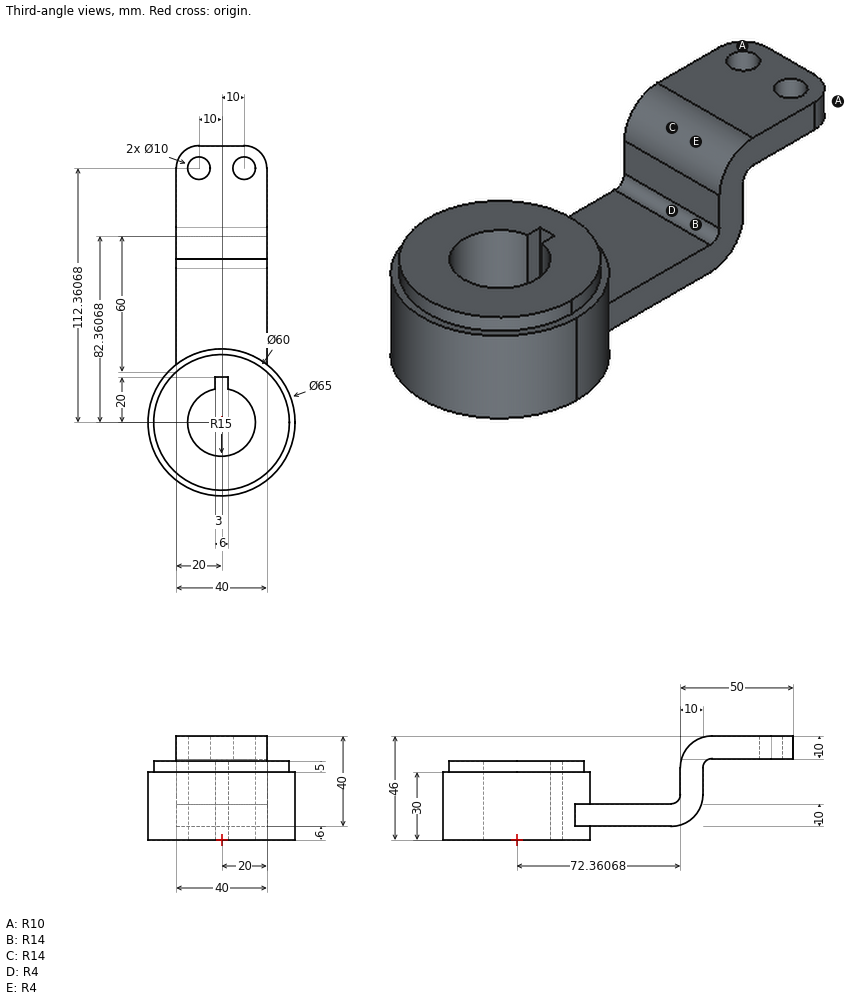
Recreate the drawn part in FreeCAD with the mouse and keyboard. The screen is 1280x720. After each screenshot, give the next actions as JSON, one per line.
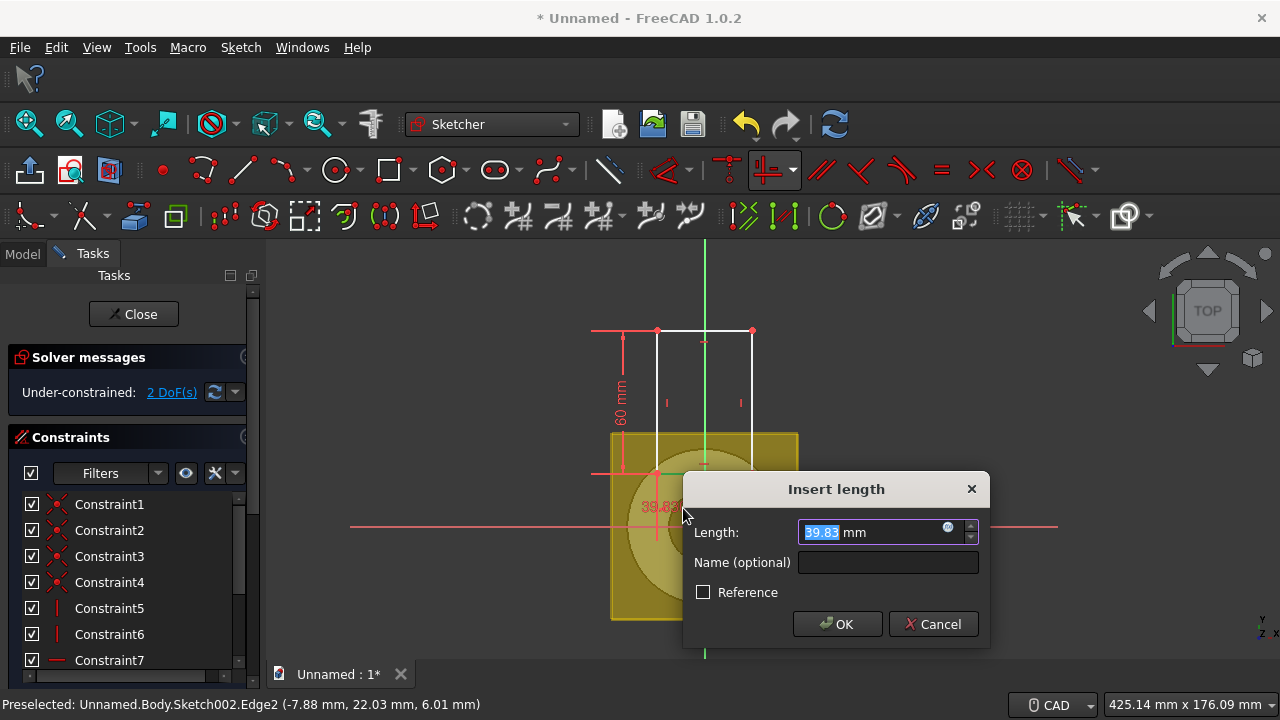
{"action": "type", "text": "40"}
{"action": "key", "text": "Return"}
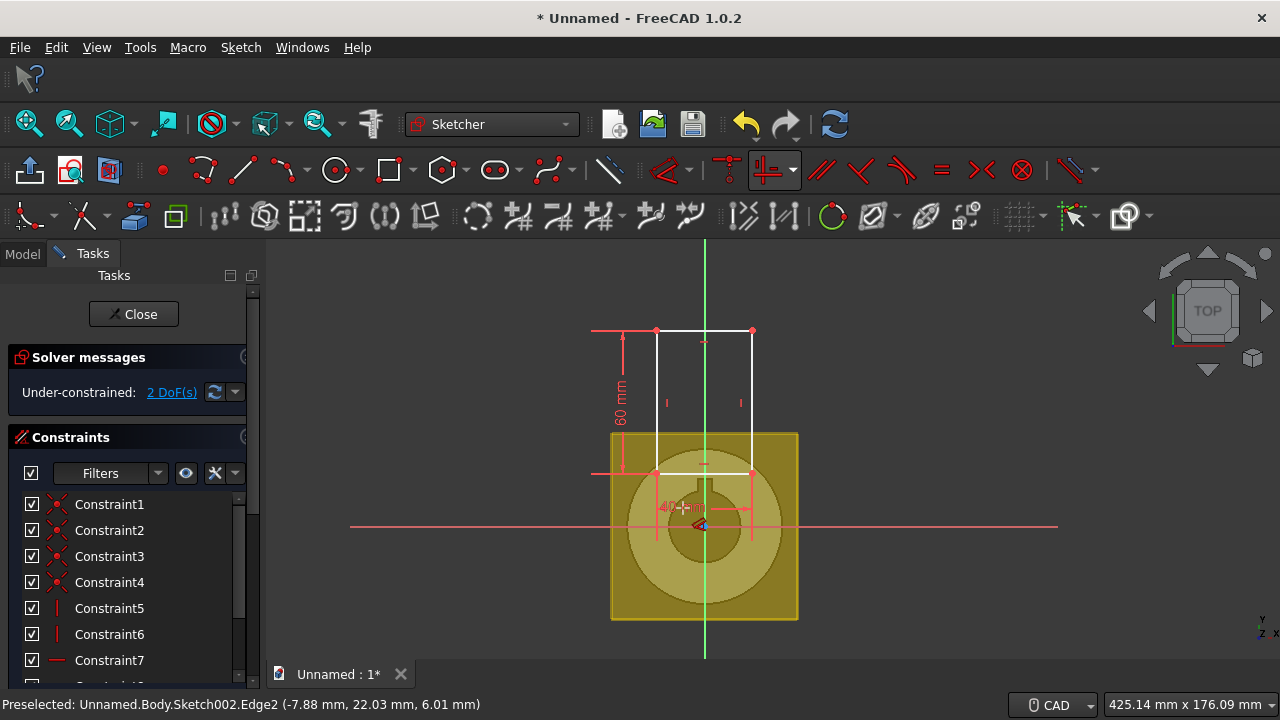
{"action": "left_click", "coordinate": [657, 331]}
{"action": "left_click", "coordinate": [681, 561]}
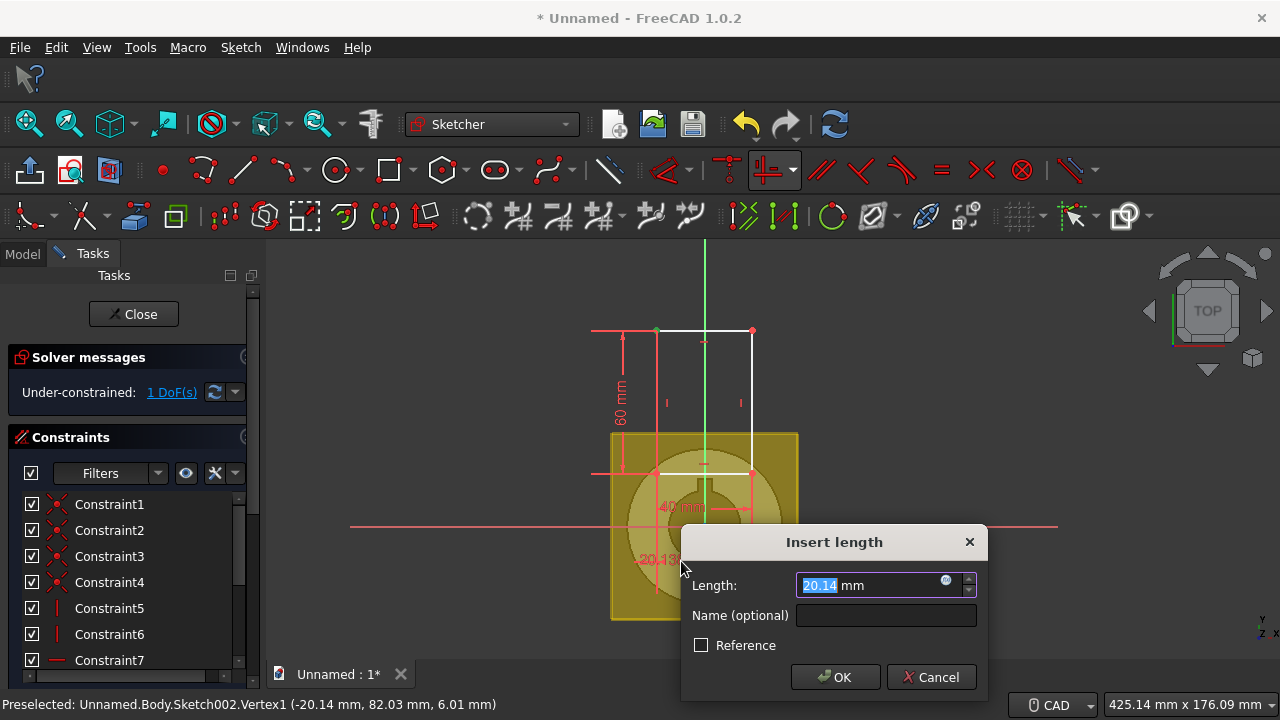
{"action": "type", "text": "20"}
{"action": "key", "text": "Return"}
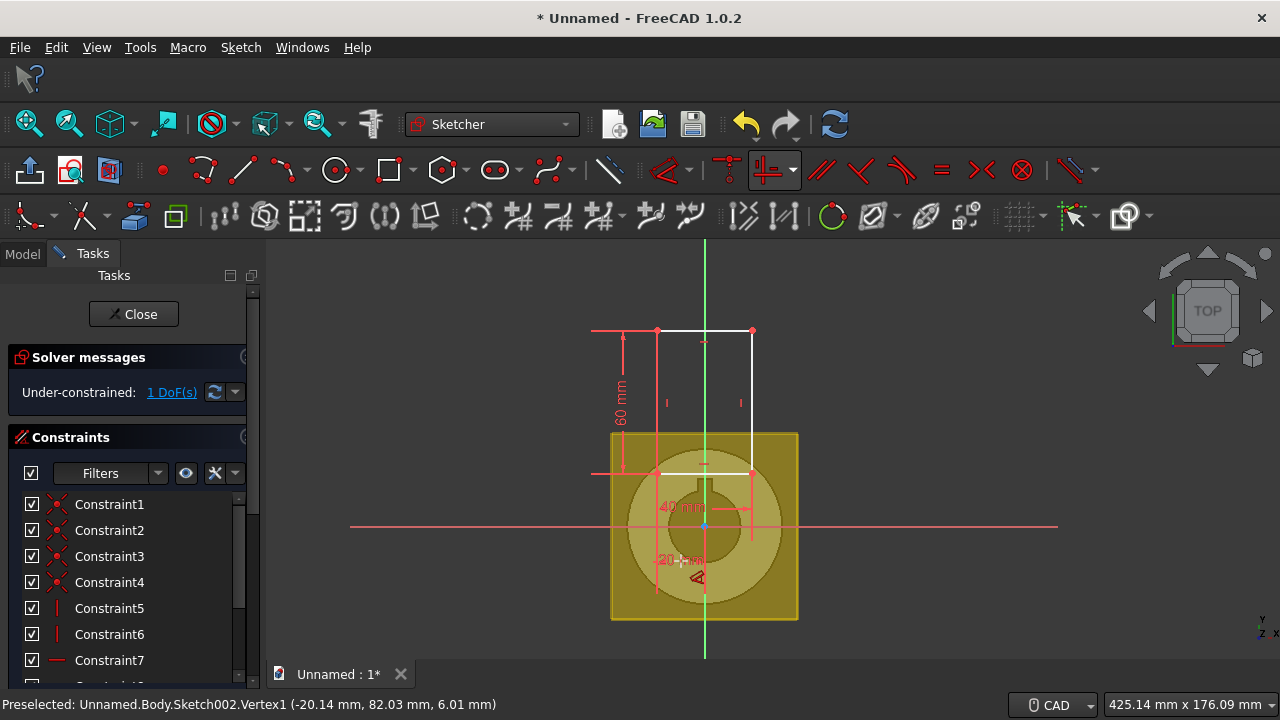
{"action": "left_click", "coordinate": [657, 331]}
{"action": "left_click", "coordinate": [623, 429]}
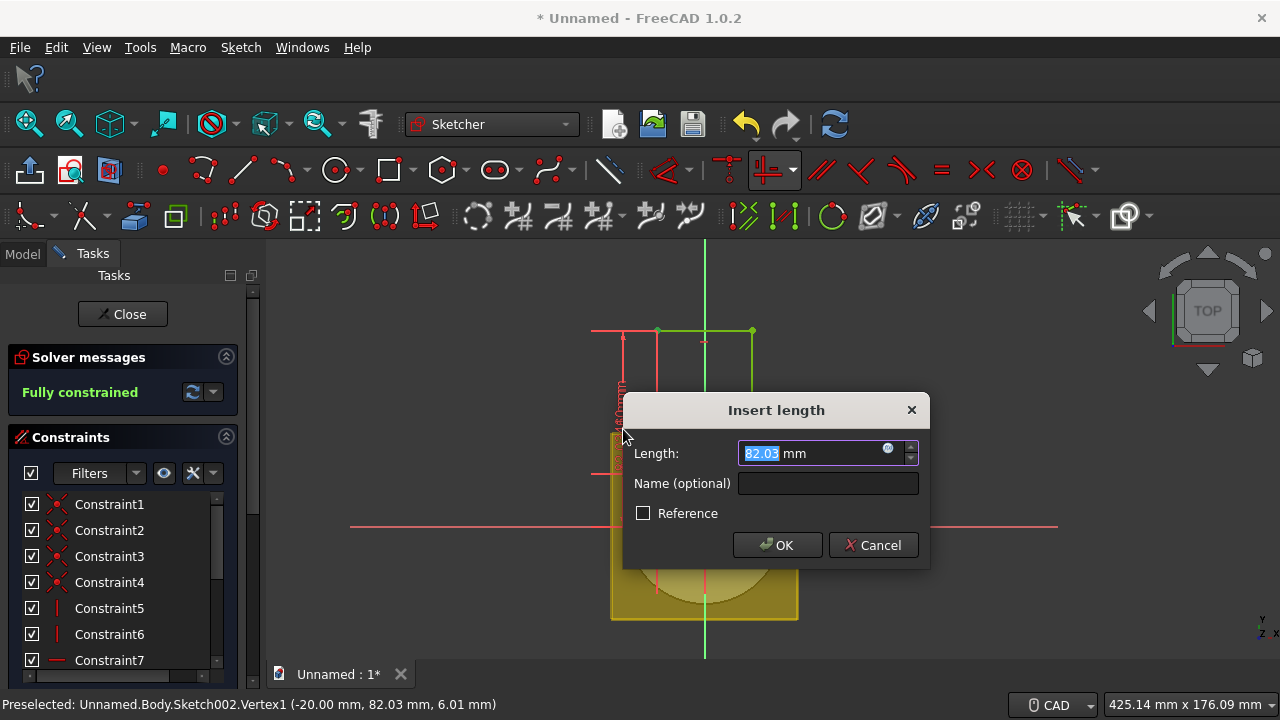
{"action": "type", "text": "82.36068"}
{"action": "key", "text": "Return"}
{"action": "key", "text": "Escape"}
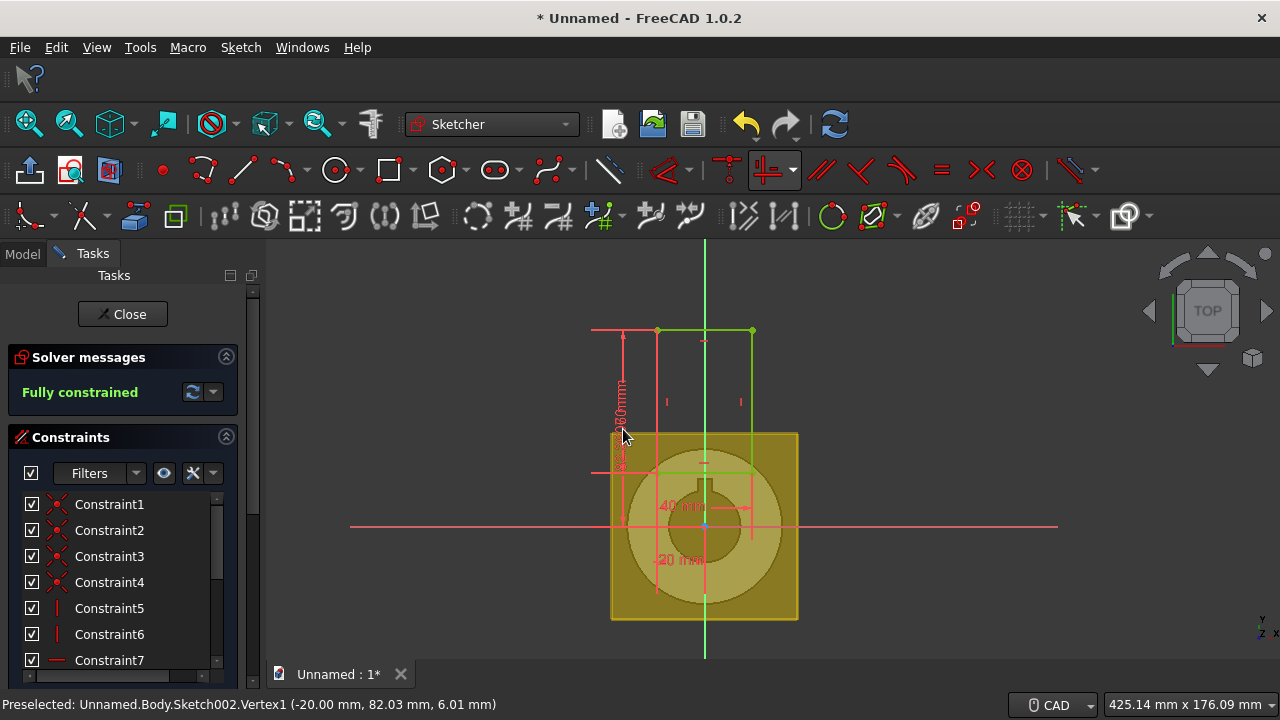
{"action": "left_click", "coordinate": [123, 314]}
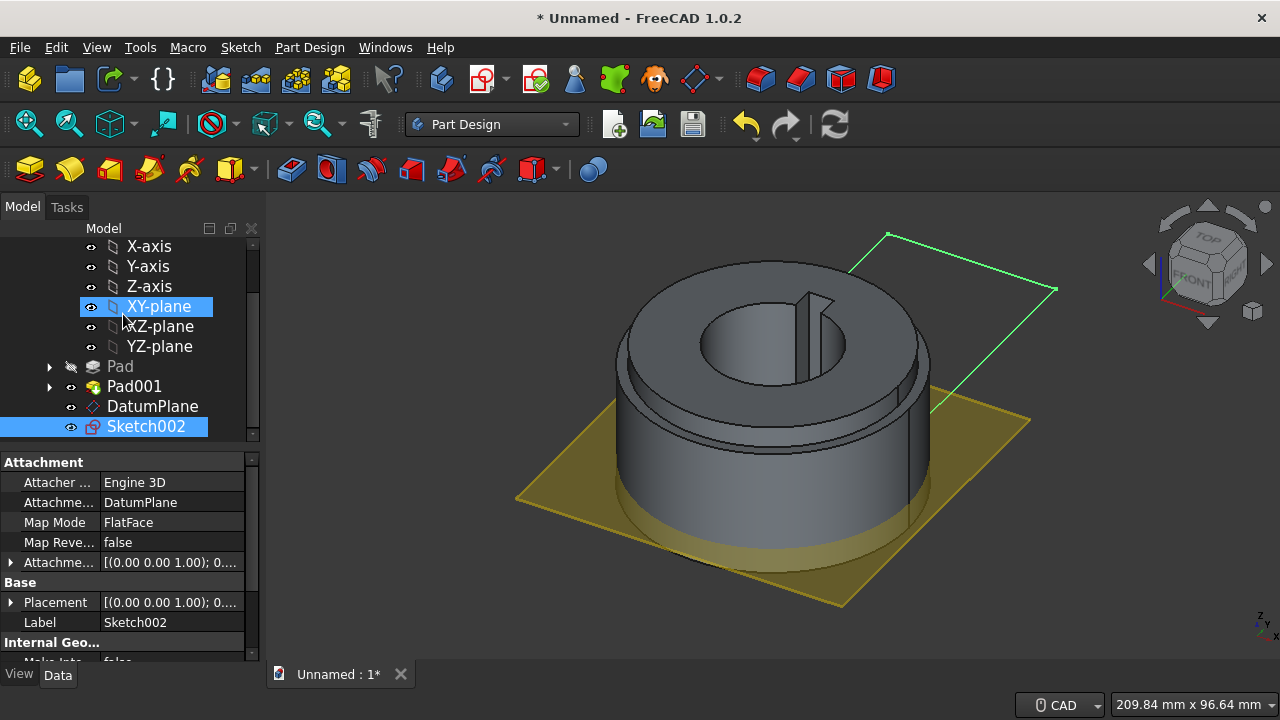
{"action": "left_click", "coordinate": [30, 170]}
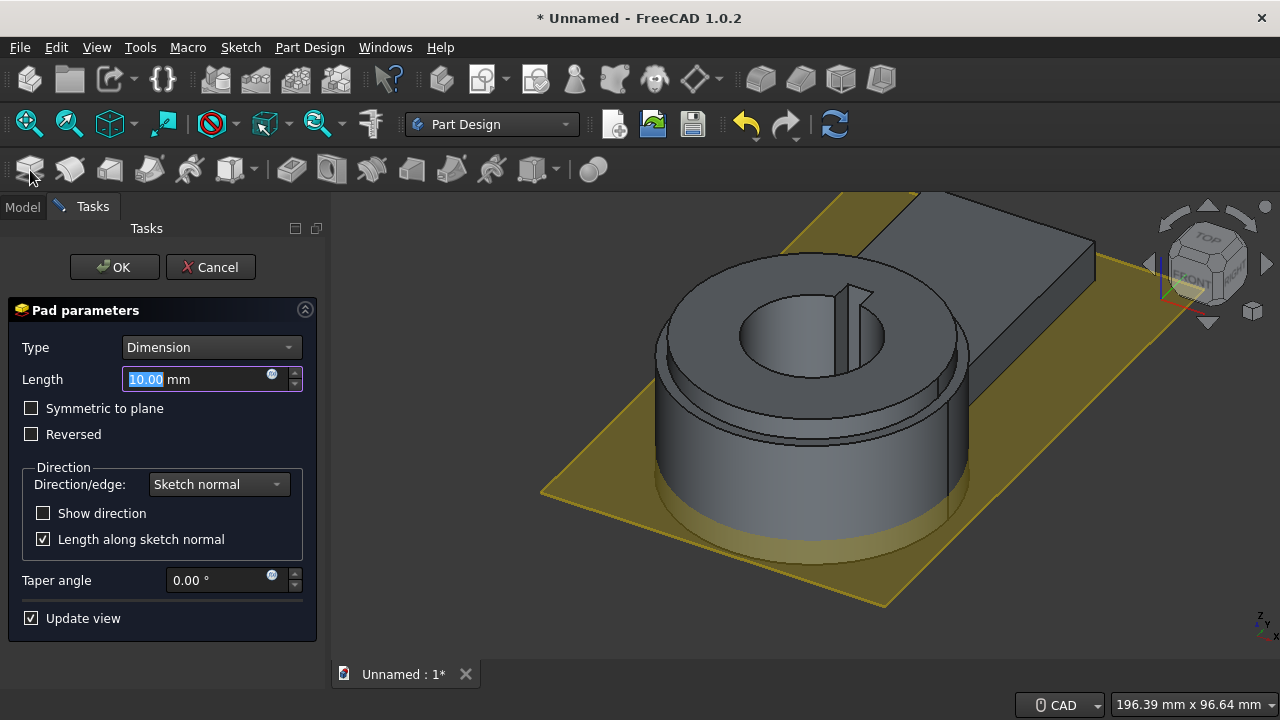
{"action": "type", "text": "10"}
{"action": "key", "text": "Tab"}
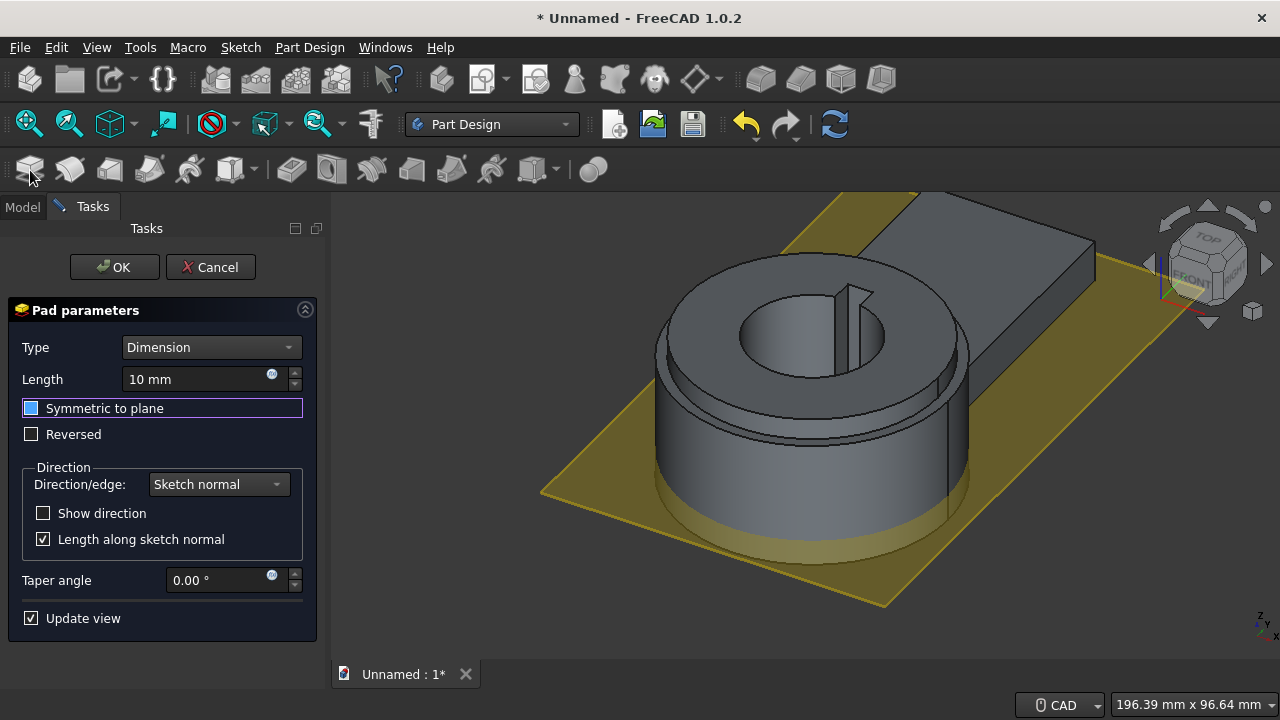
{"action": "left_click", "coordinate": [115, 267]}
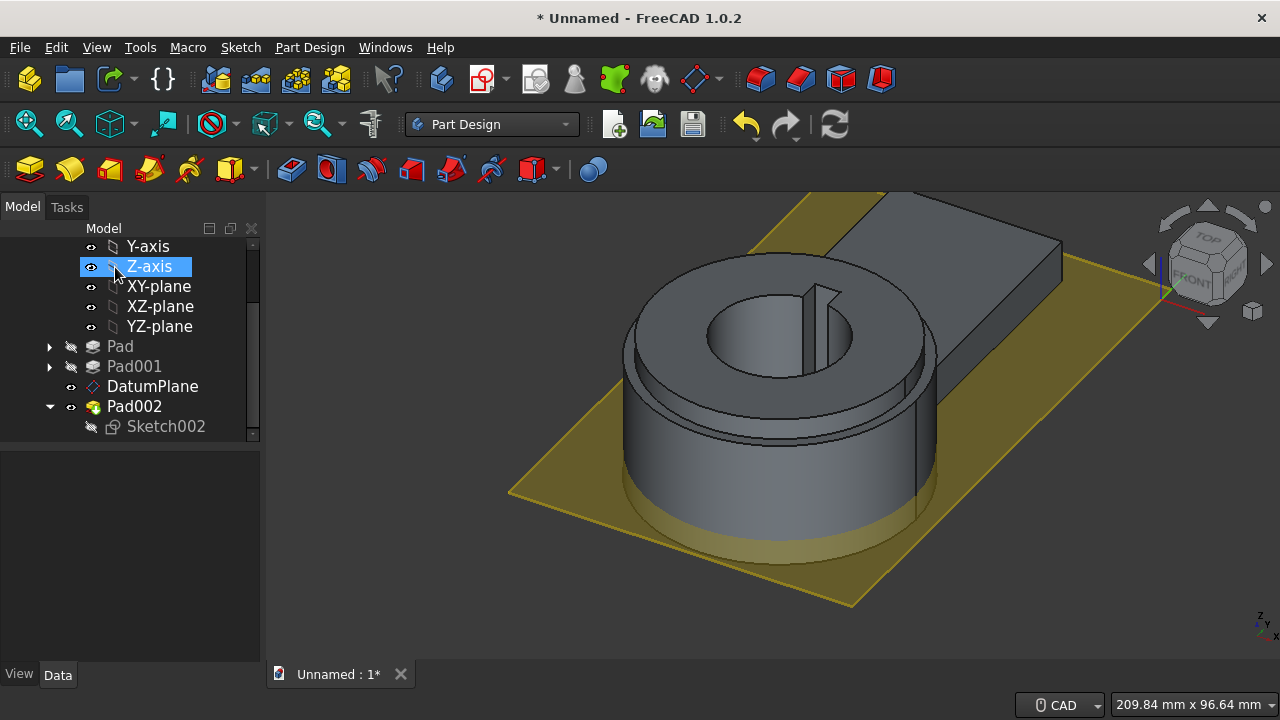
{"action": "left_click", "coordinate": [116, 387]}
{"action": "key", "text": "space"}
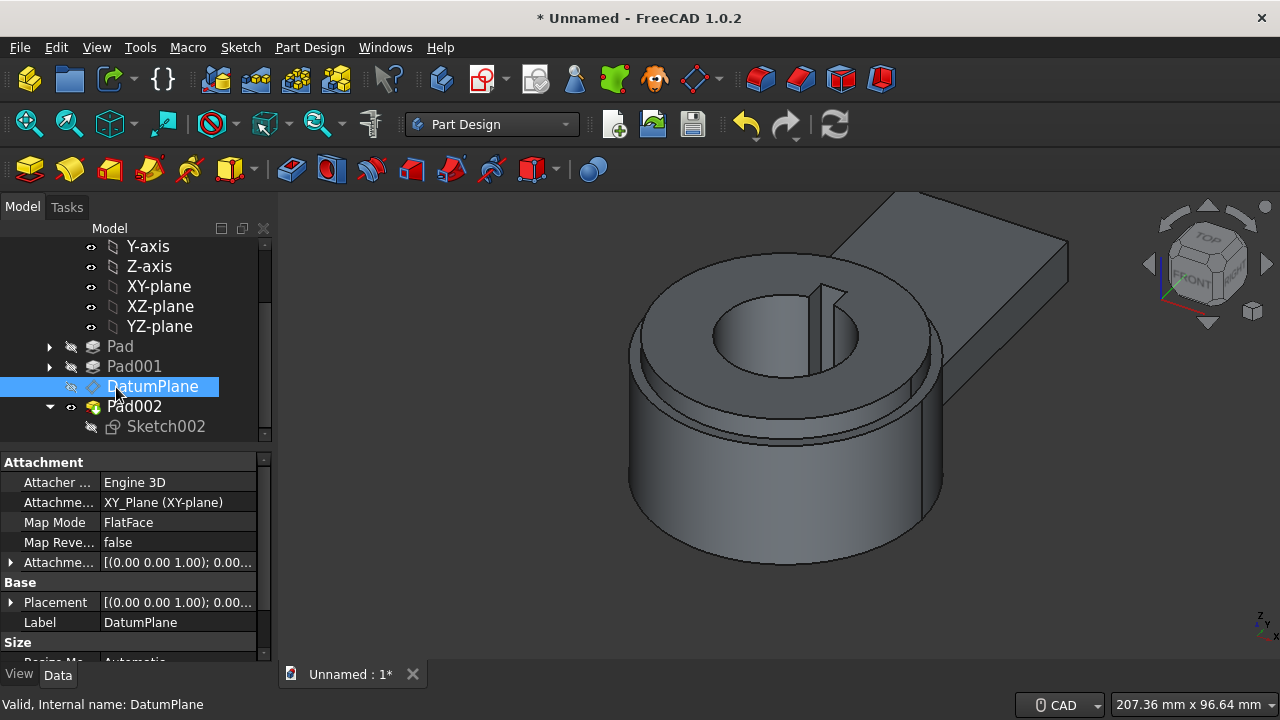
{"action": "key", "text": "v f"}